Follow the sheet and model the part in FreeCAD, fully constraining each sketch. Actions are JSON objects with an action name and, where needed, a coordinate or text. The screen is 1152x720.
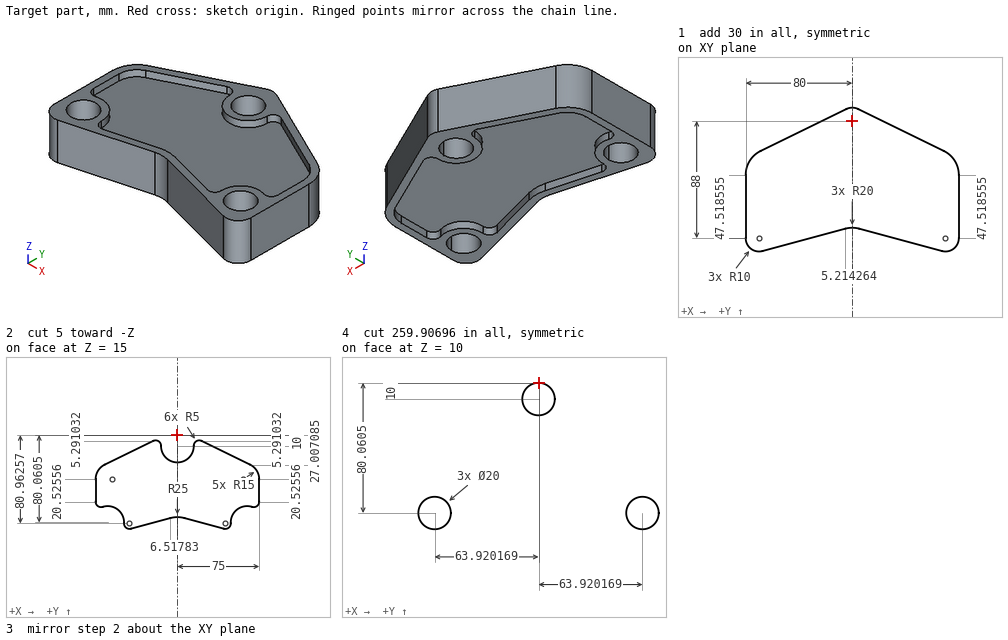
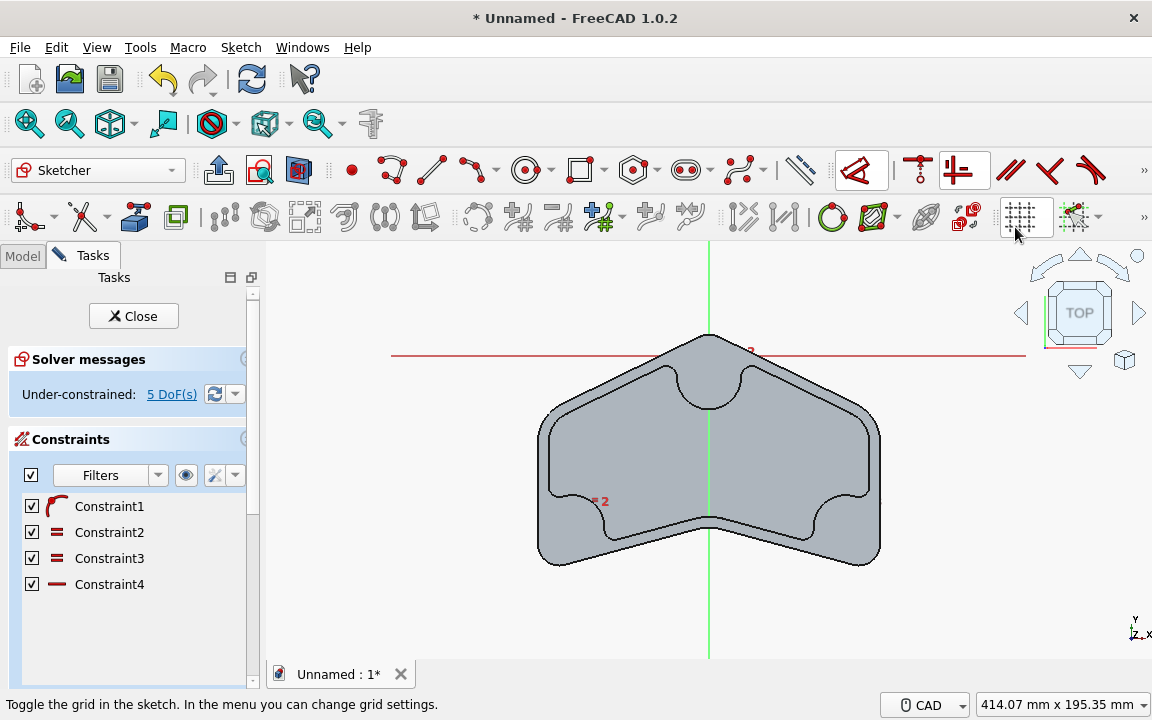
{"action": "left_click", "coordinate": [588, 513]}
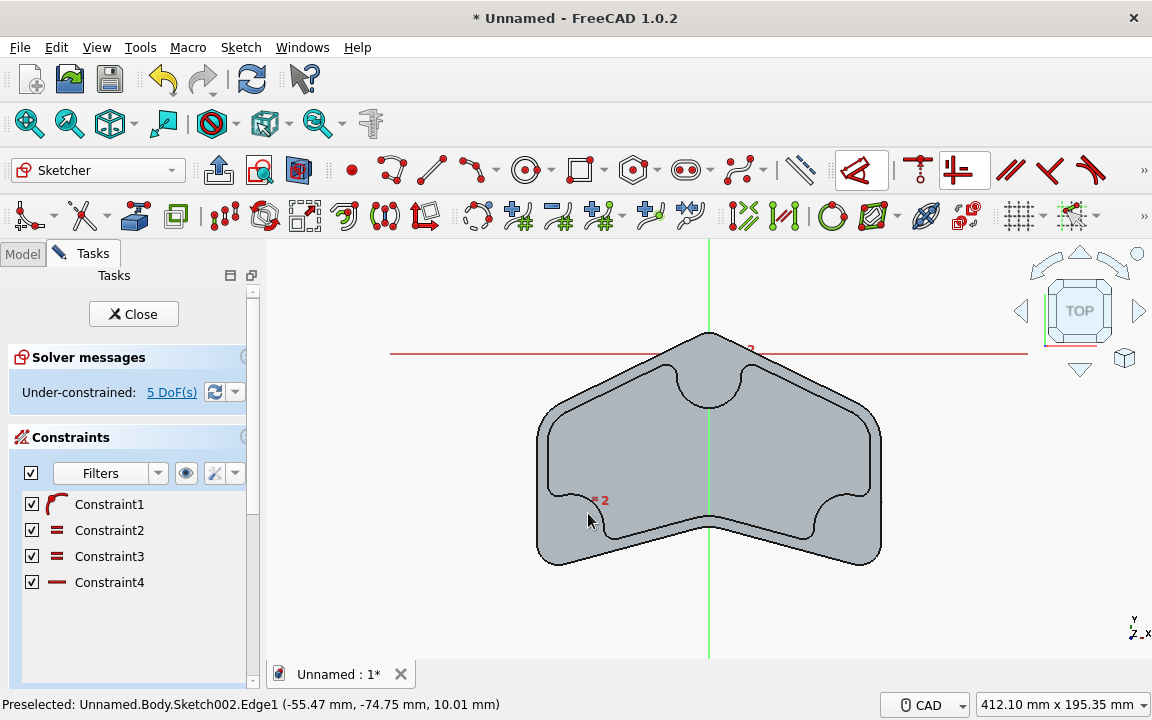
{"action": "left_click", "coordinate": [882, 170]}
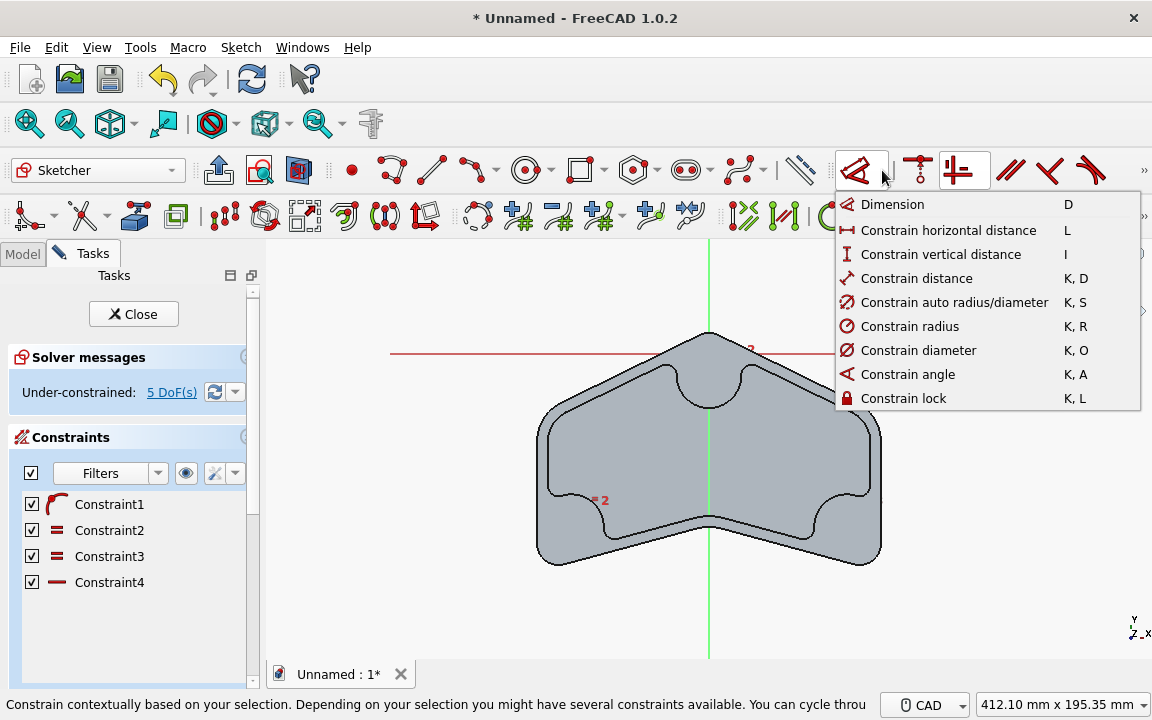
{"action": "left_click", "coordinate": [988, 350]}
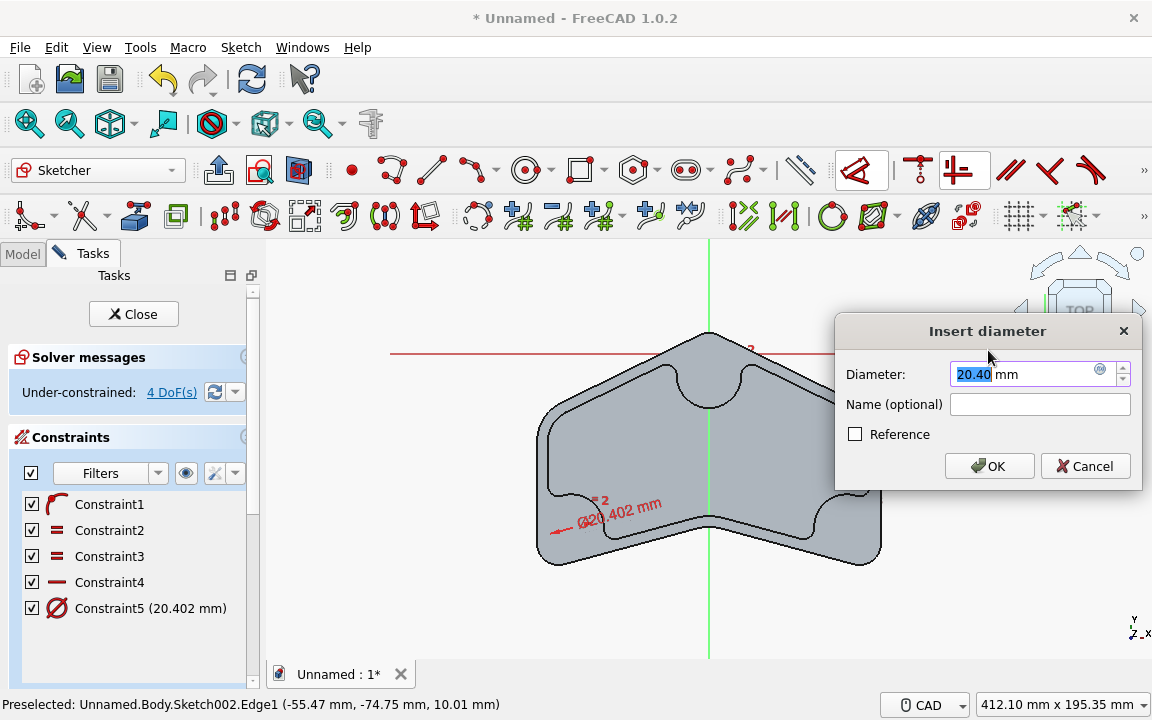
{"action": "type", "text": "20"}
{"action": "key", "text": "Return"}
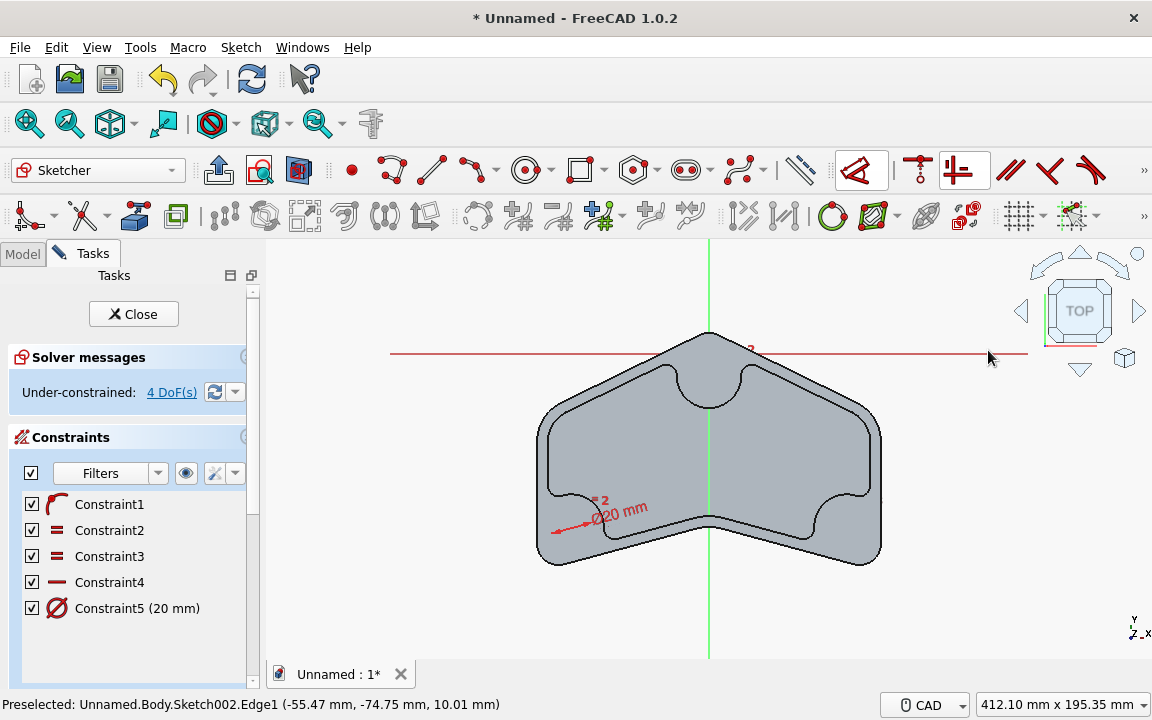
{"action": "scroll", "coordinate": [709, 377], "scroll_direction": "up", "scroll_amount": 4}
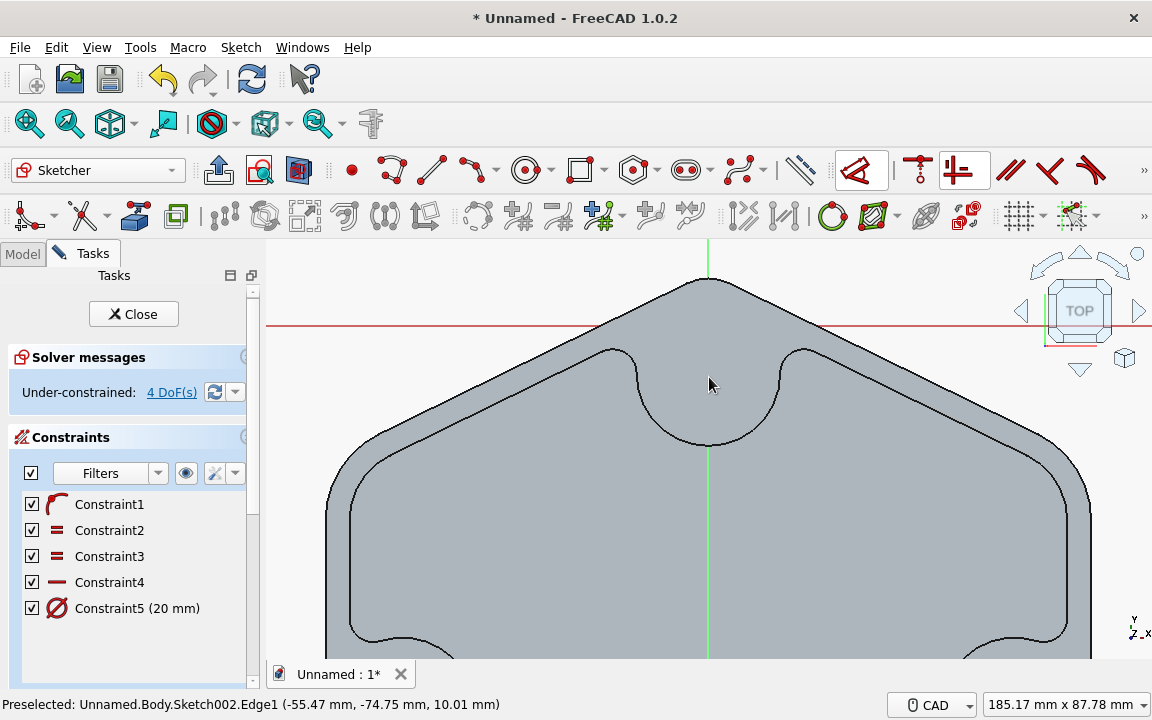
{"action": "left_click", "coordinate": [708, 377]}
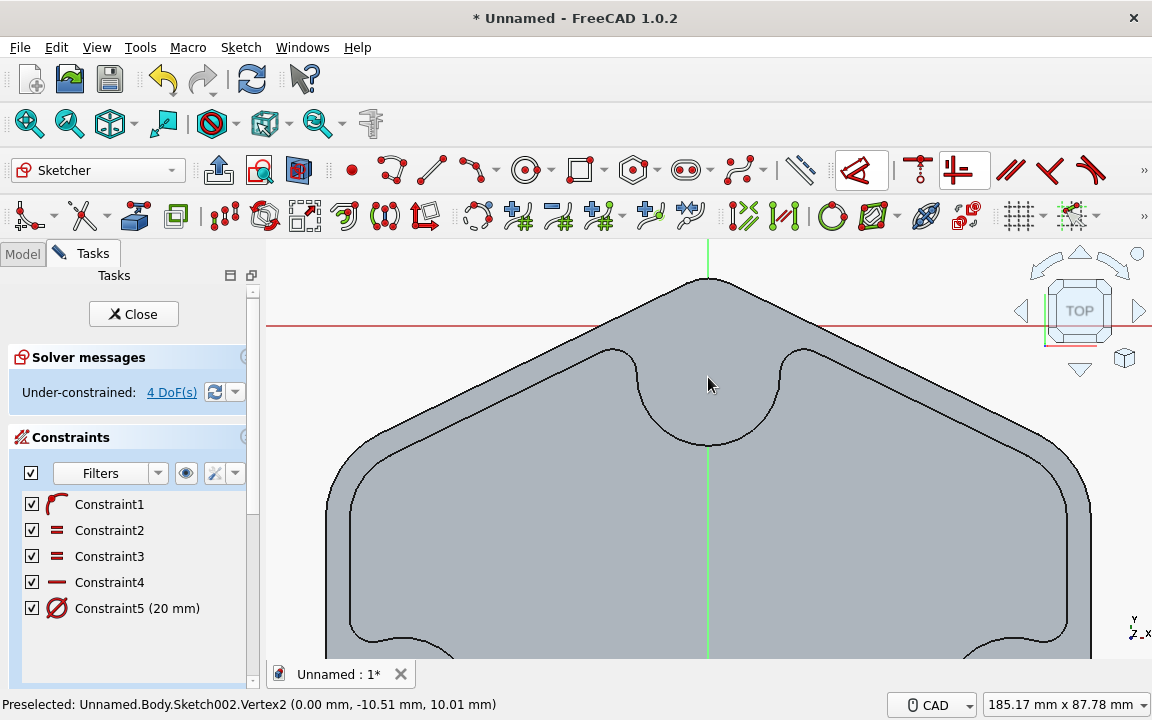
{"action": "left_click", "coordinate": [882, 170]}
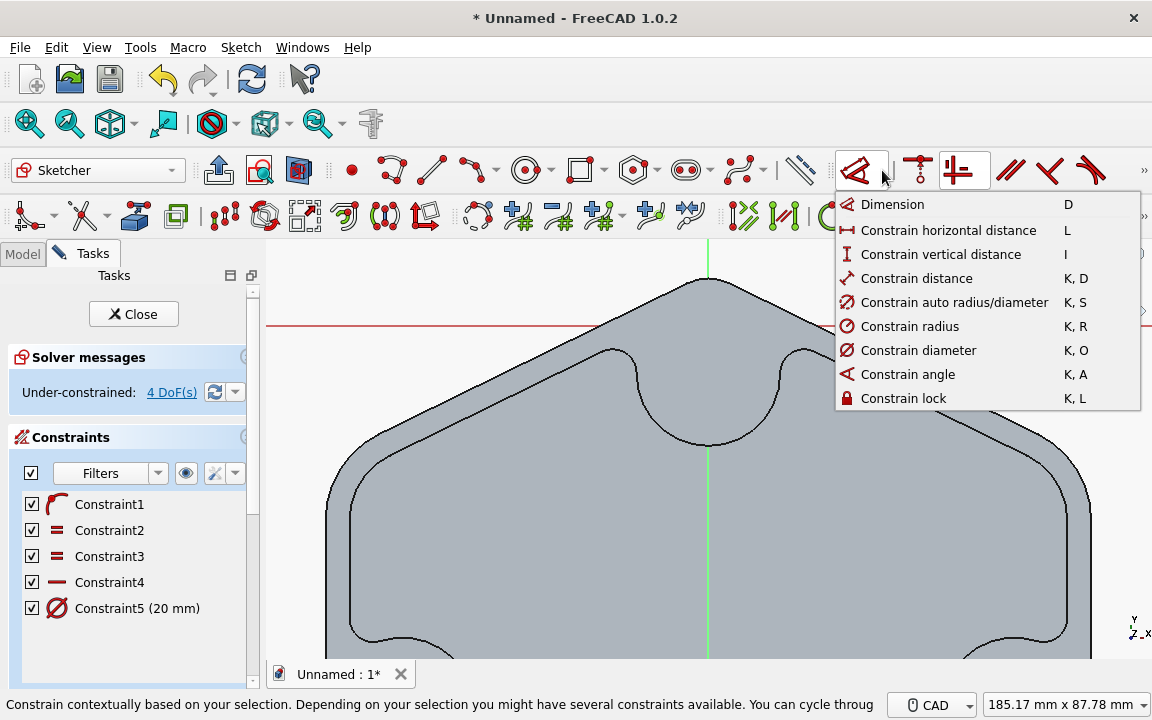
{"action": "left_click", "coordinate": [988, 254]}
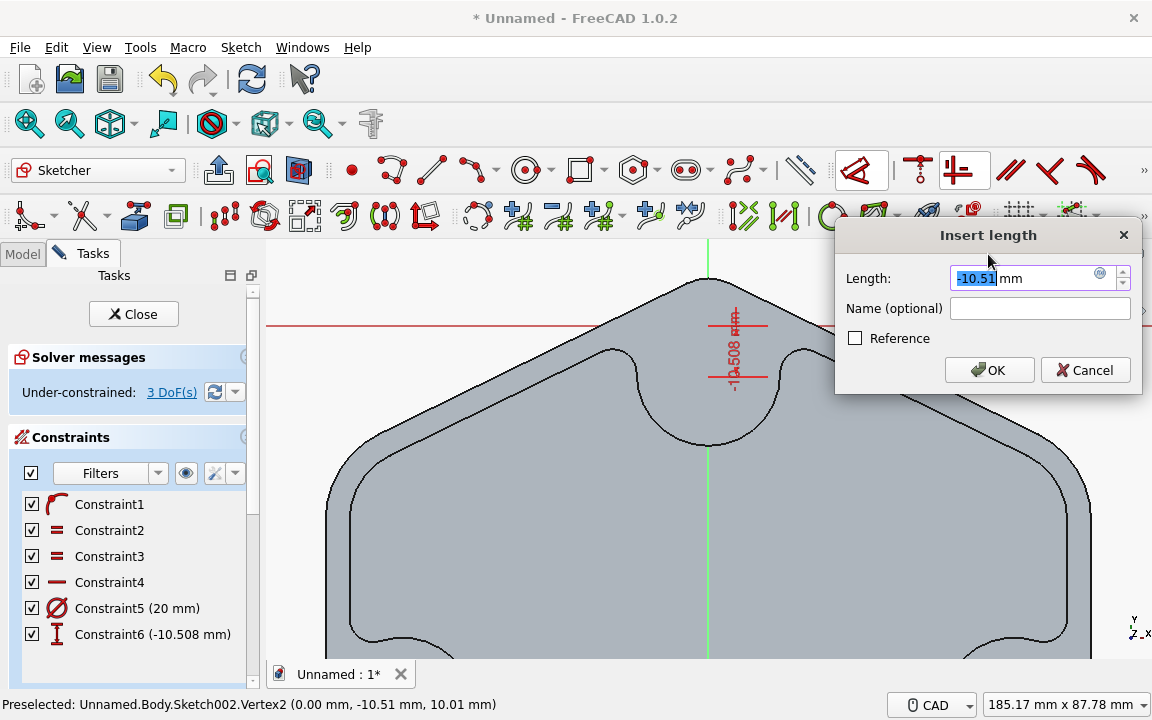
{"action": "type", "text": "-10"}
{"action": "key", "text": "Return"}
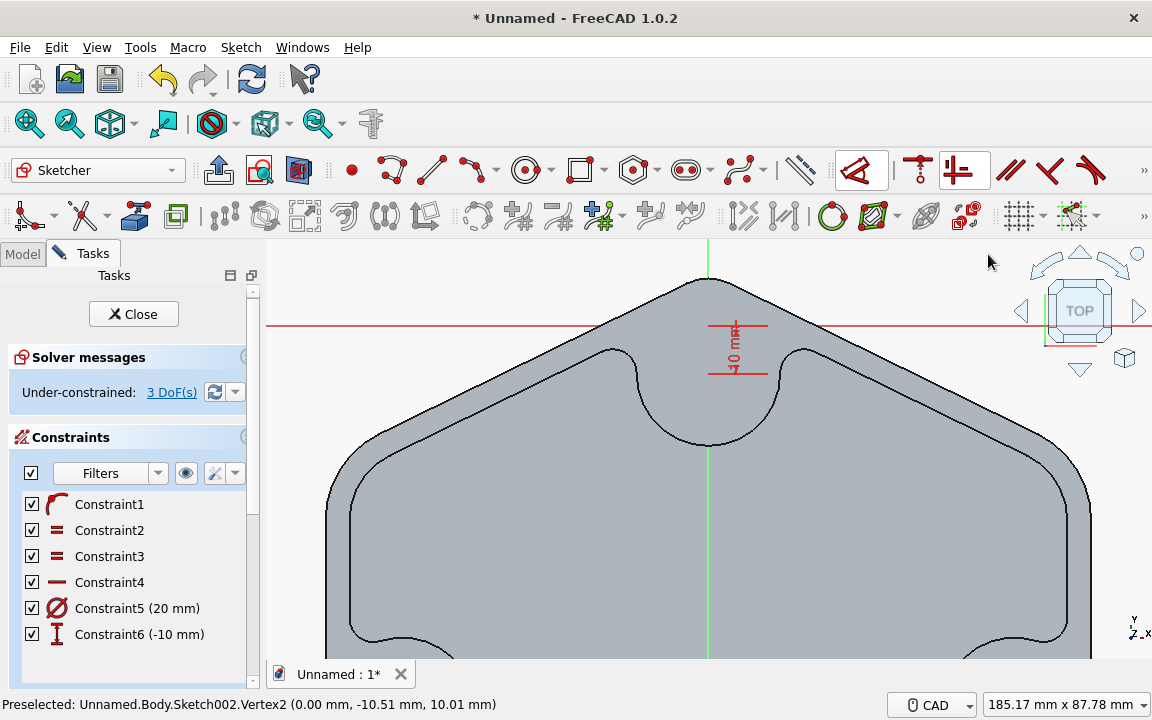
{"action": "scroll", "coordinate": [558, 336], "scroll_direction": "down", "scroll_amount": 3}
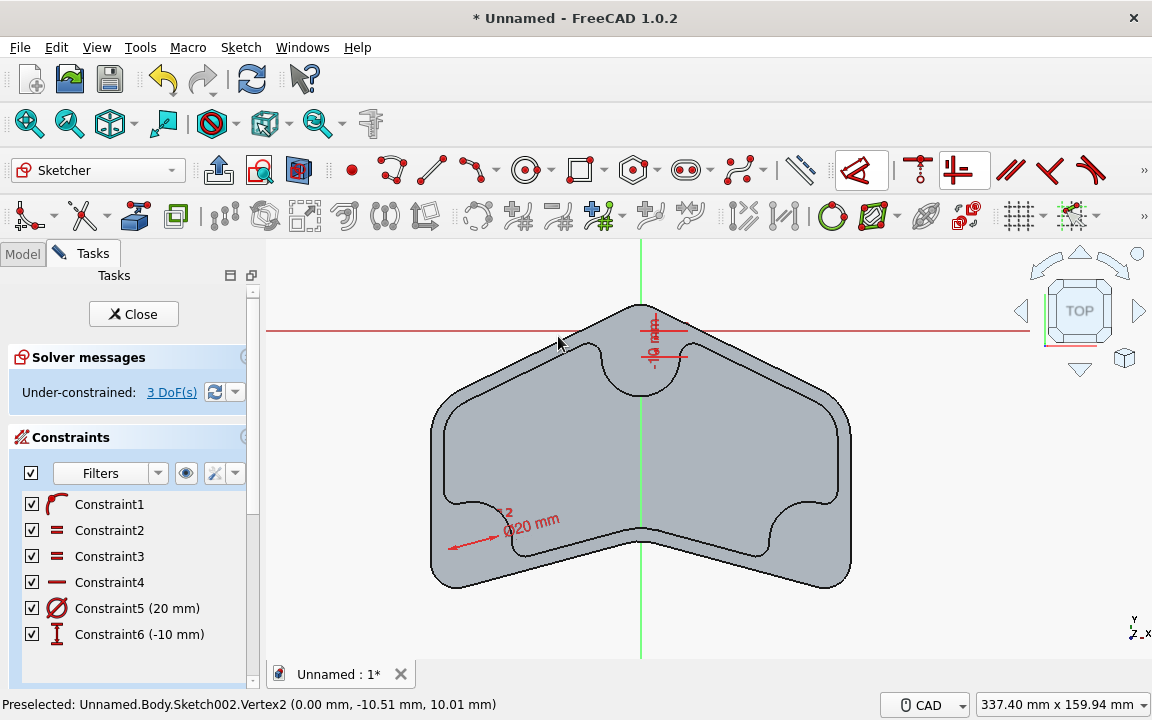
{"action": "left_click", "coordinate": [473, 543]}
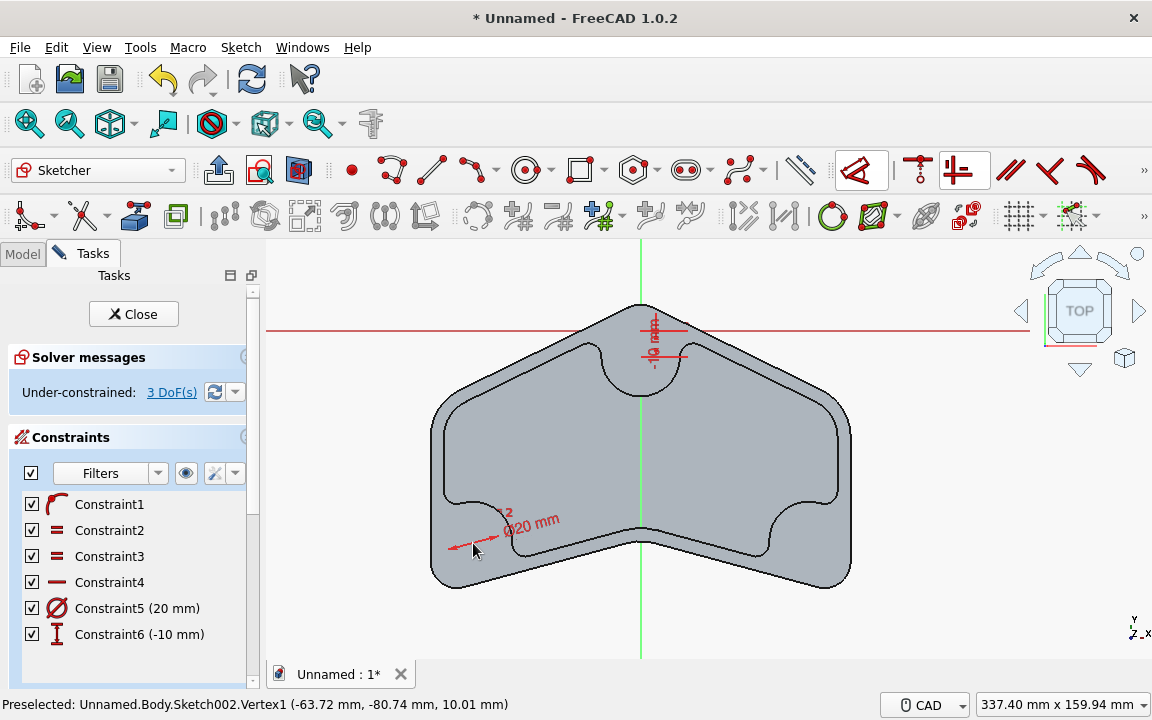
{"action": "left_click", "coordinate": [882, 170]}